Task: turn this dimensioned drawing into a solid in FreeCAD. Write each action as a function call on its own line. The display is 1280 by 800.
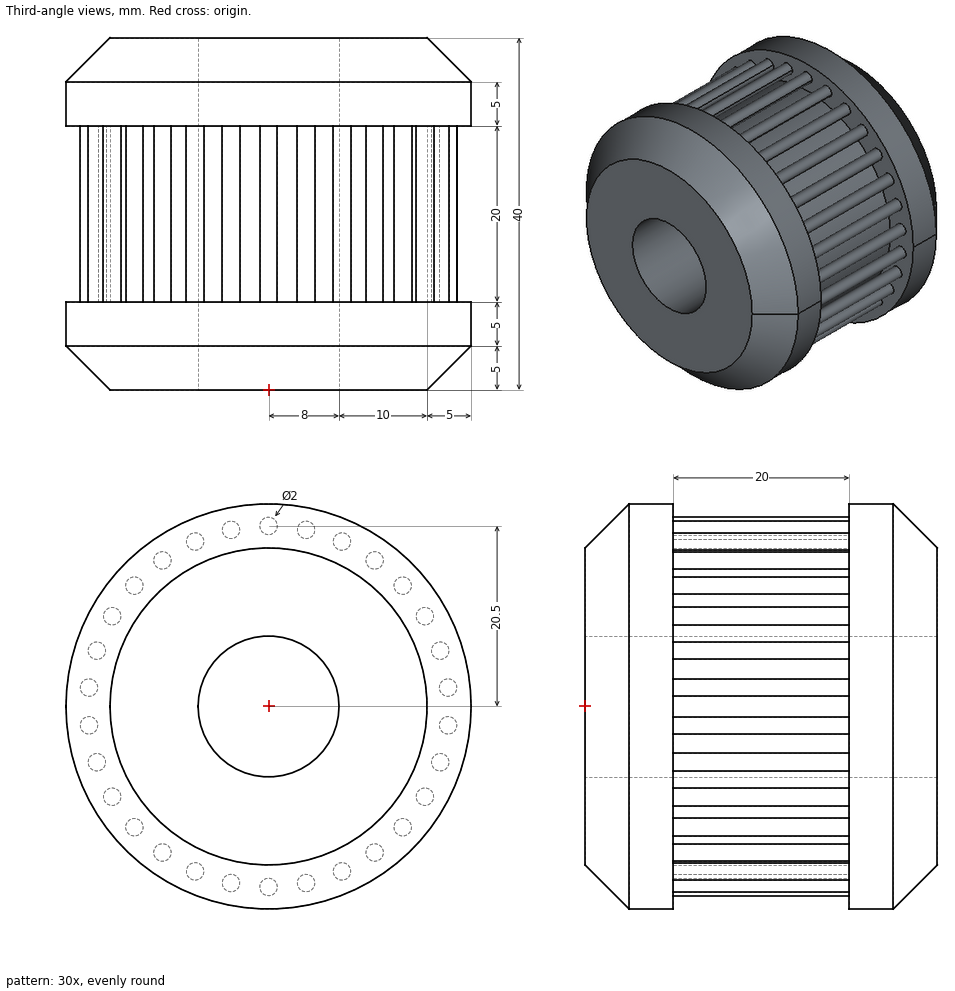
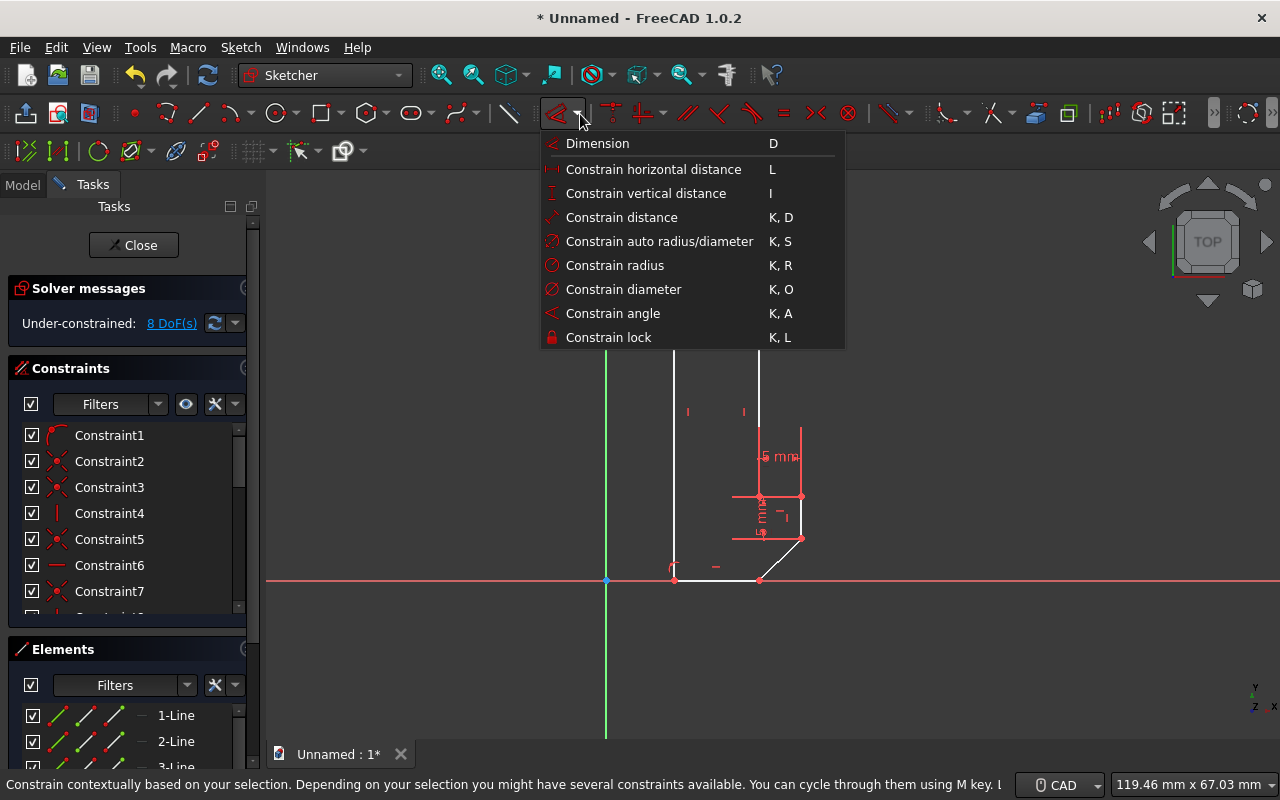
click(693, 193)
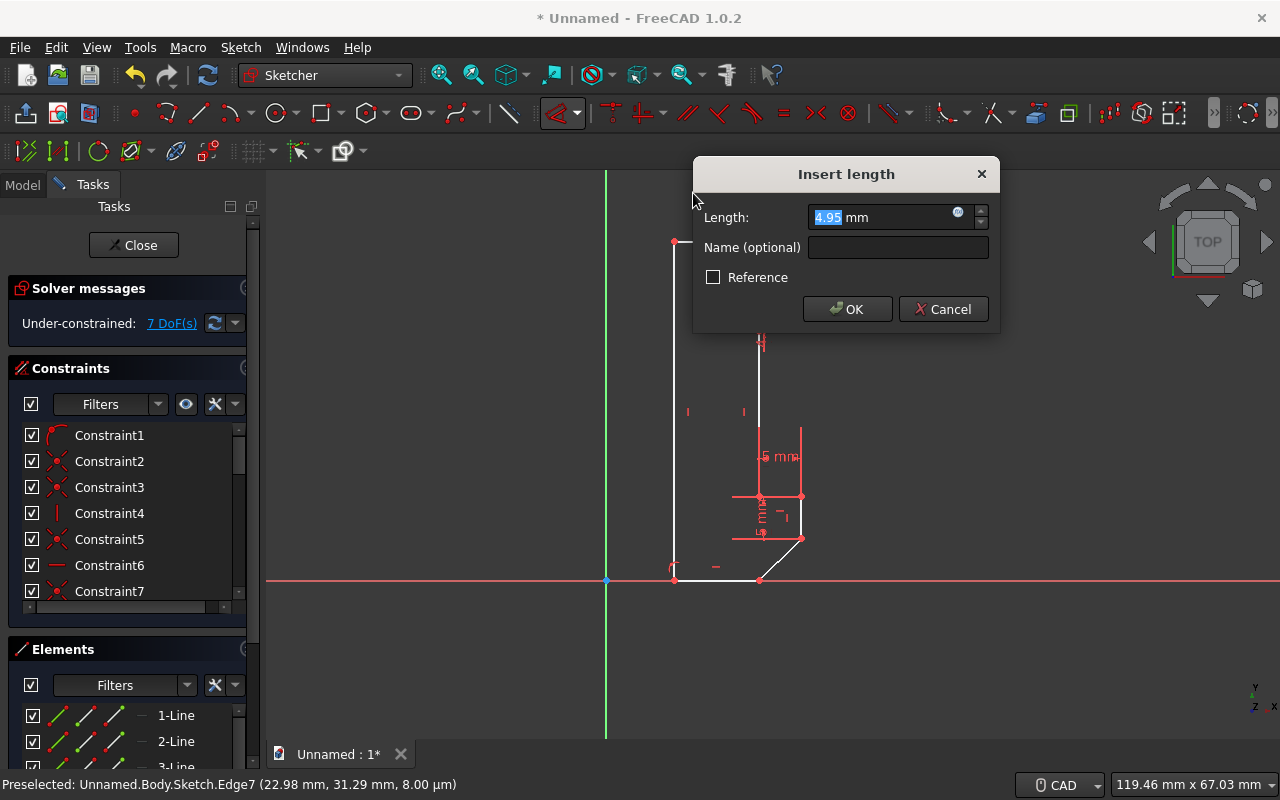
text(5)
key(Return)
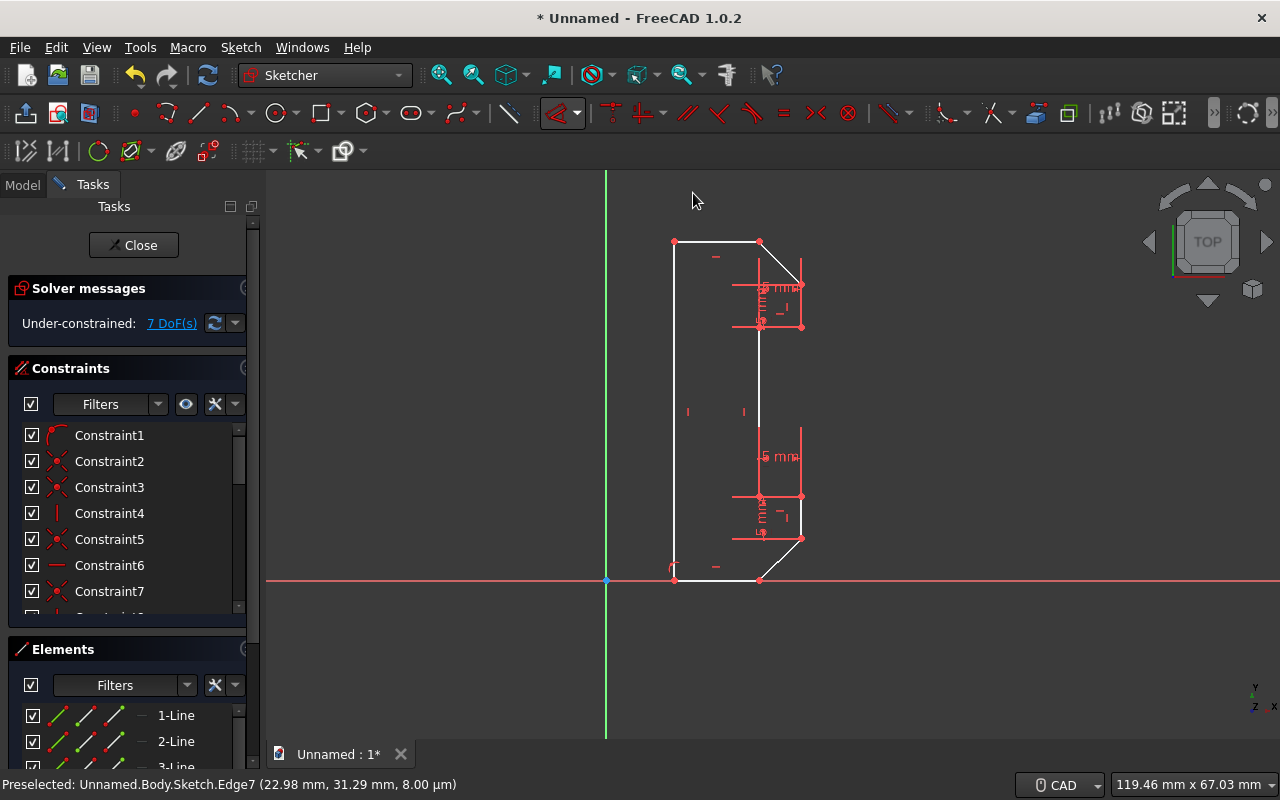
click(700, 581)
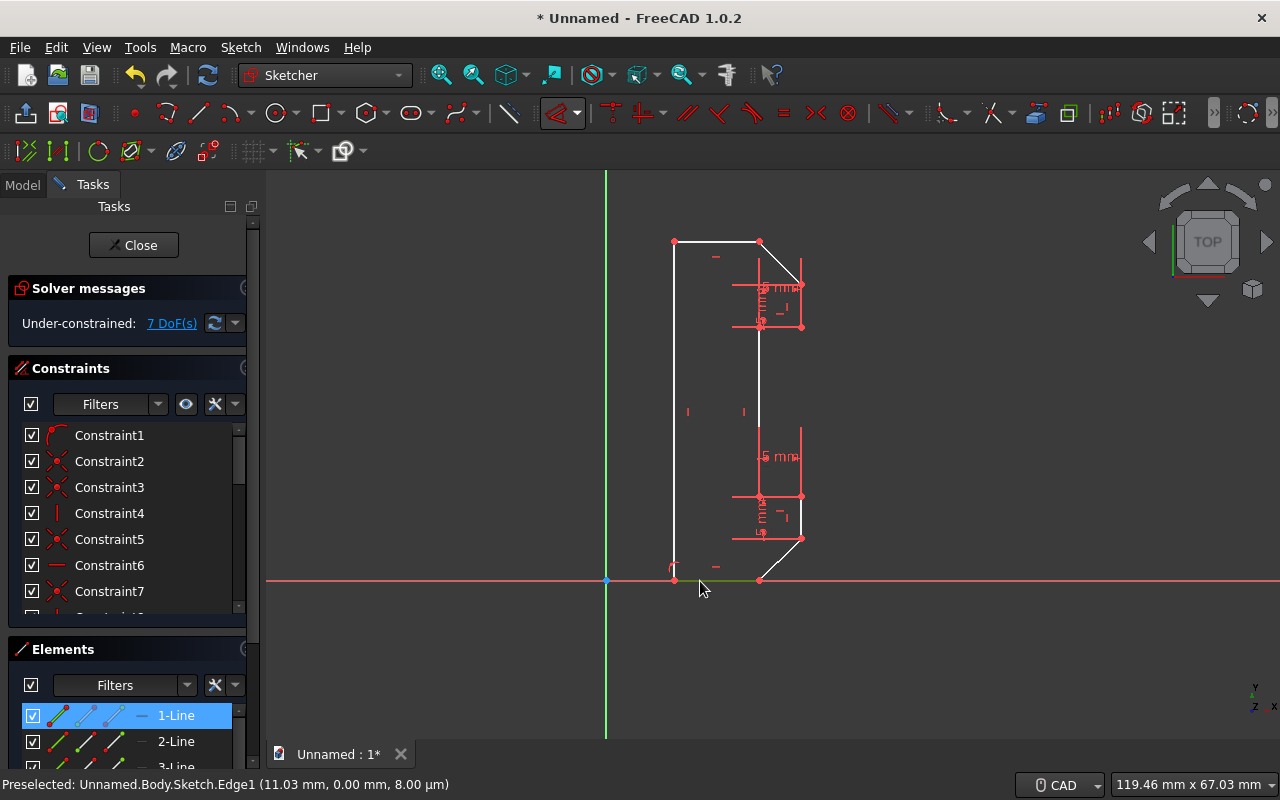
click(580, 114)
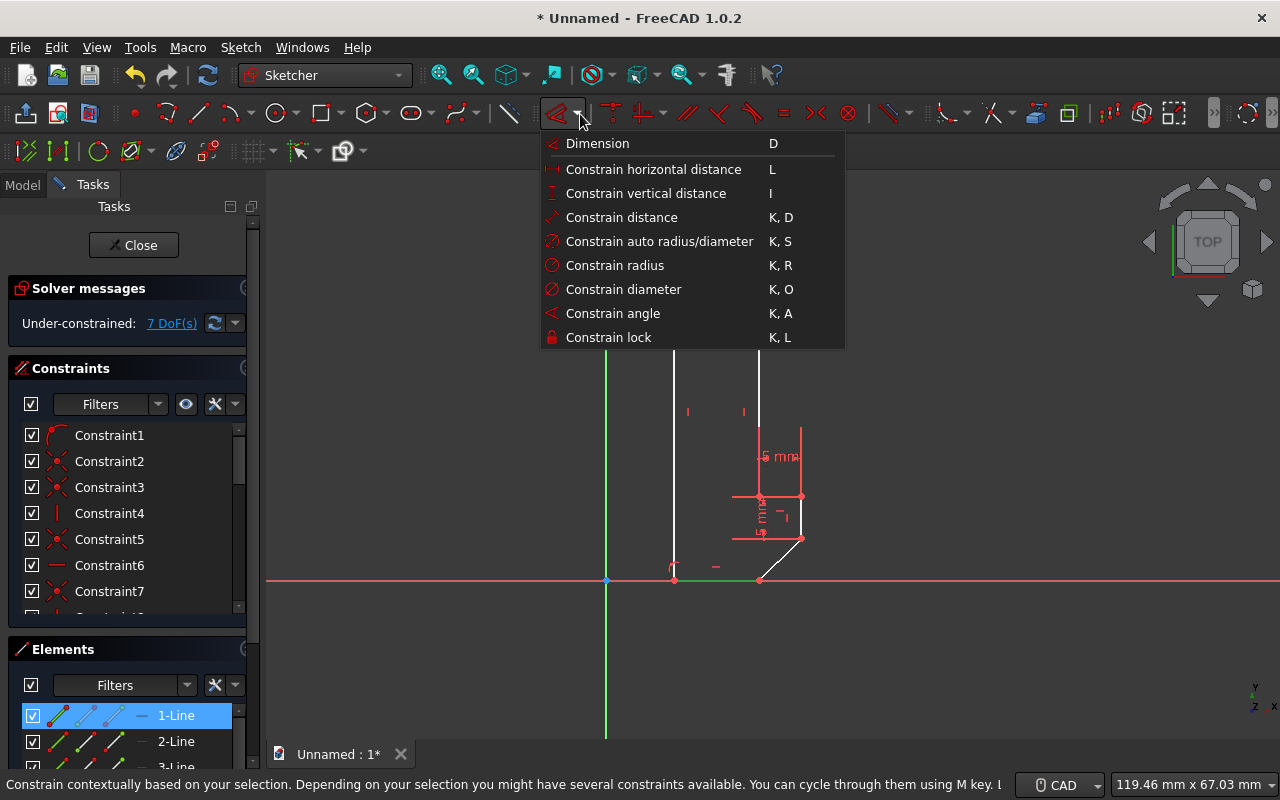
click(693, 169)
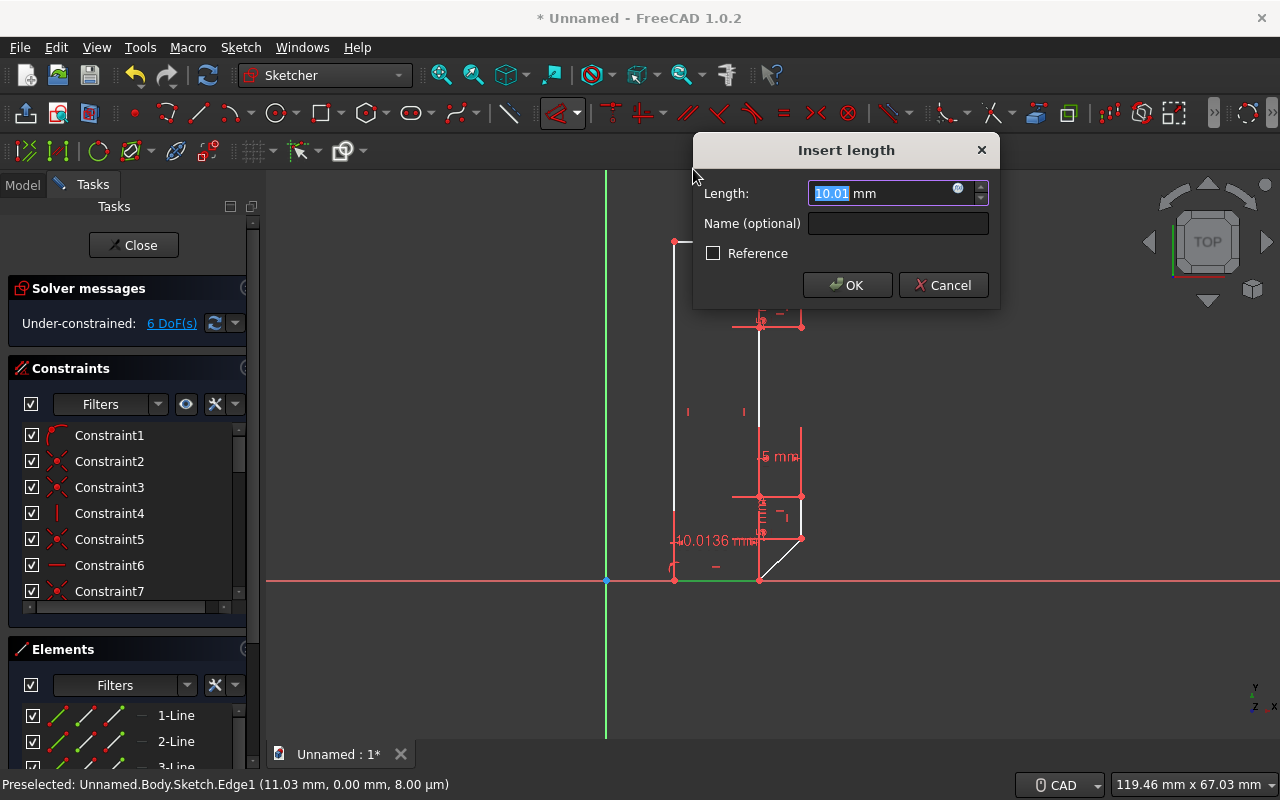
text(10)
key(Return)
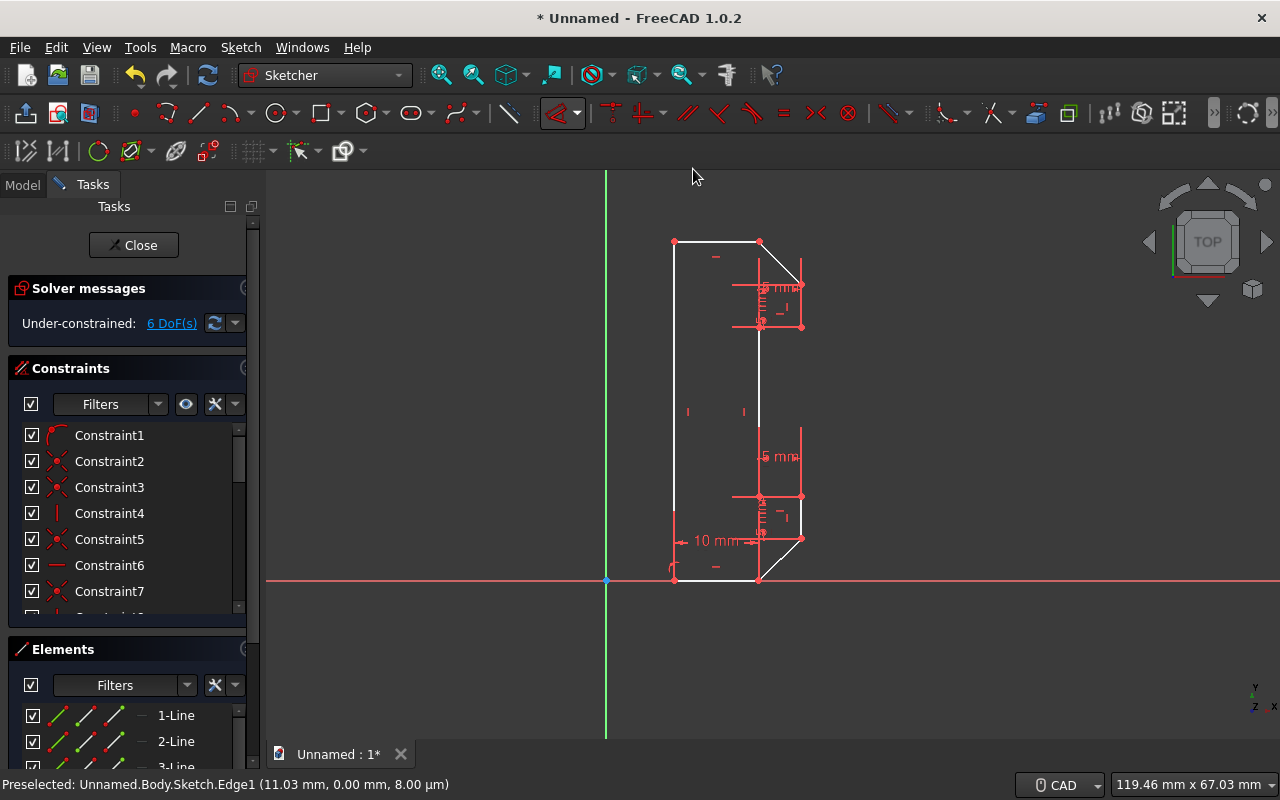
click(759, 446)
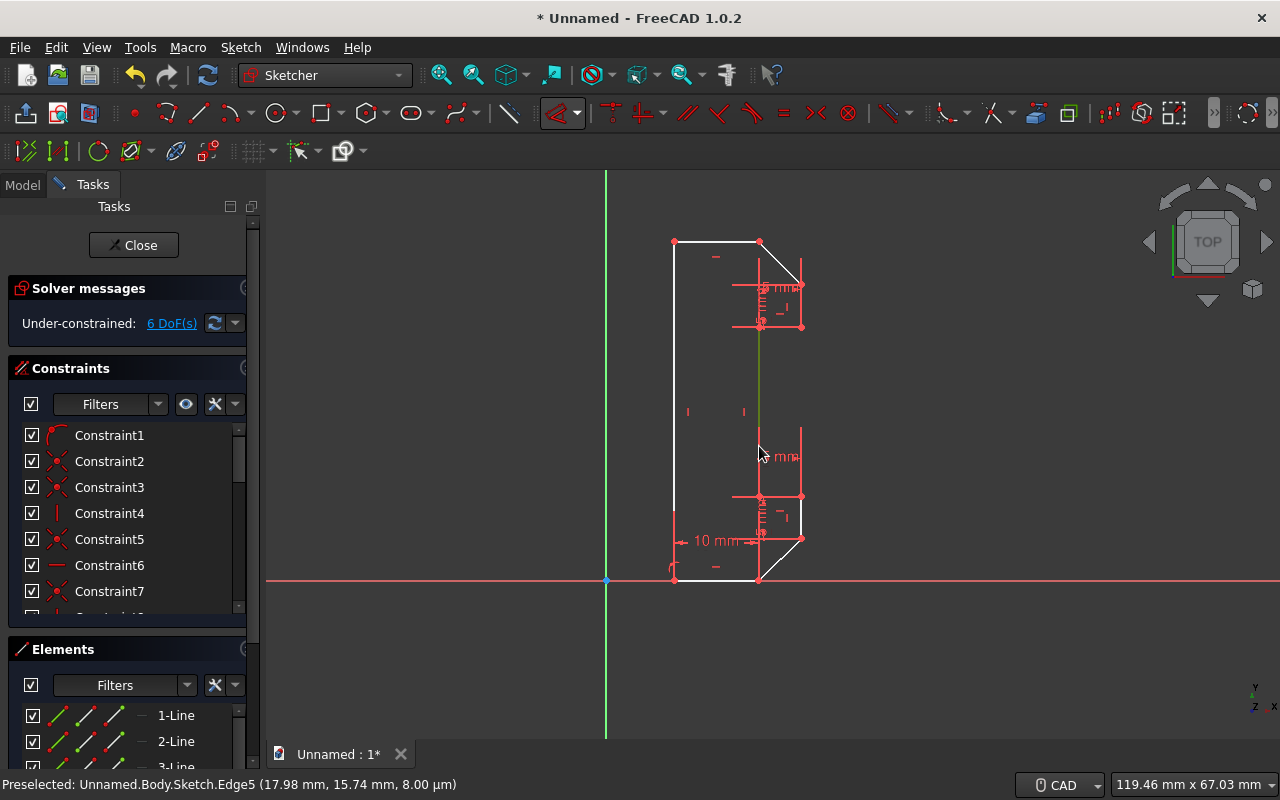
key(i)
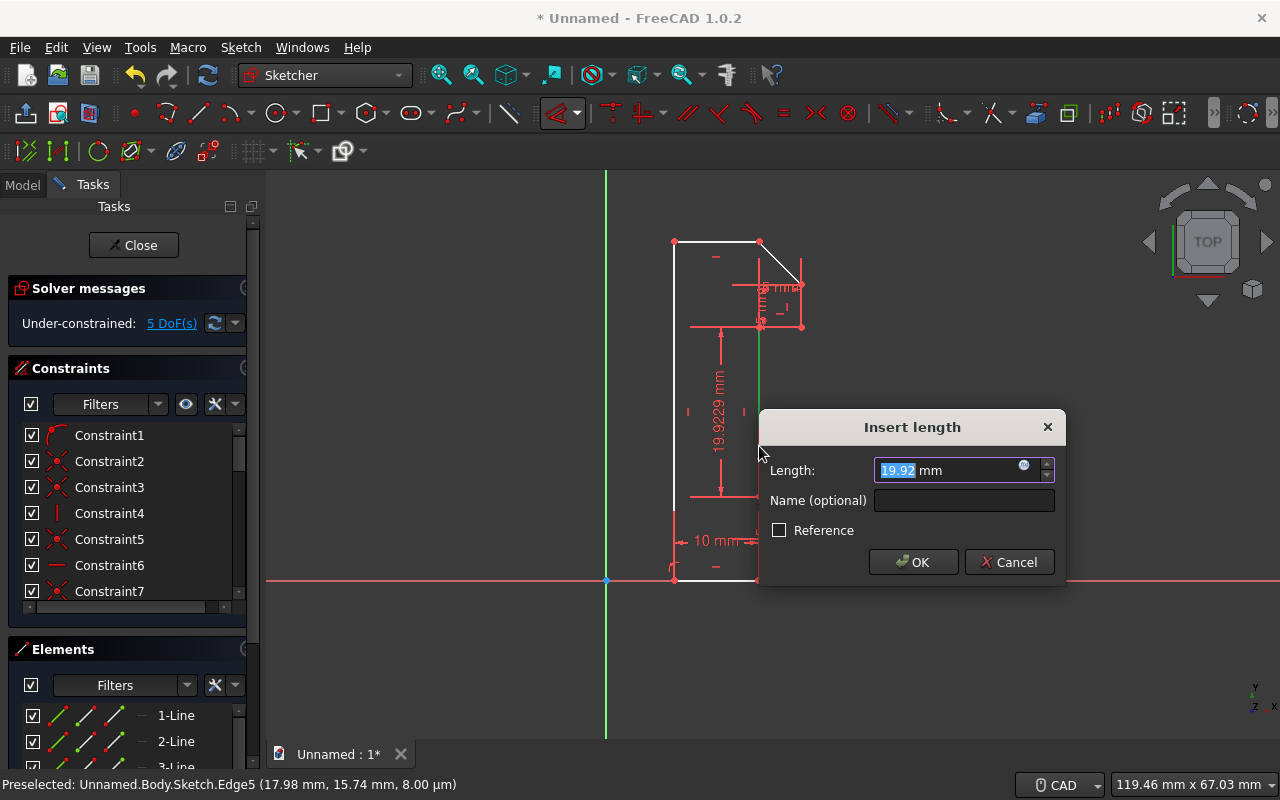
text(20)
key(Return)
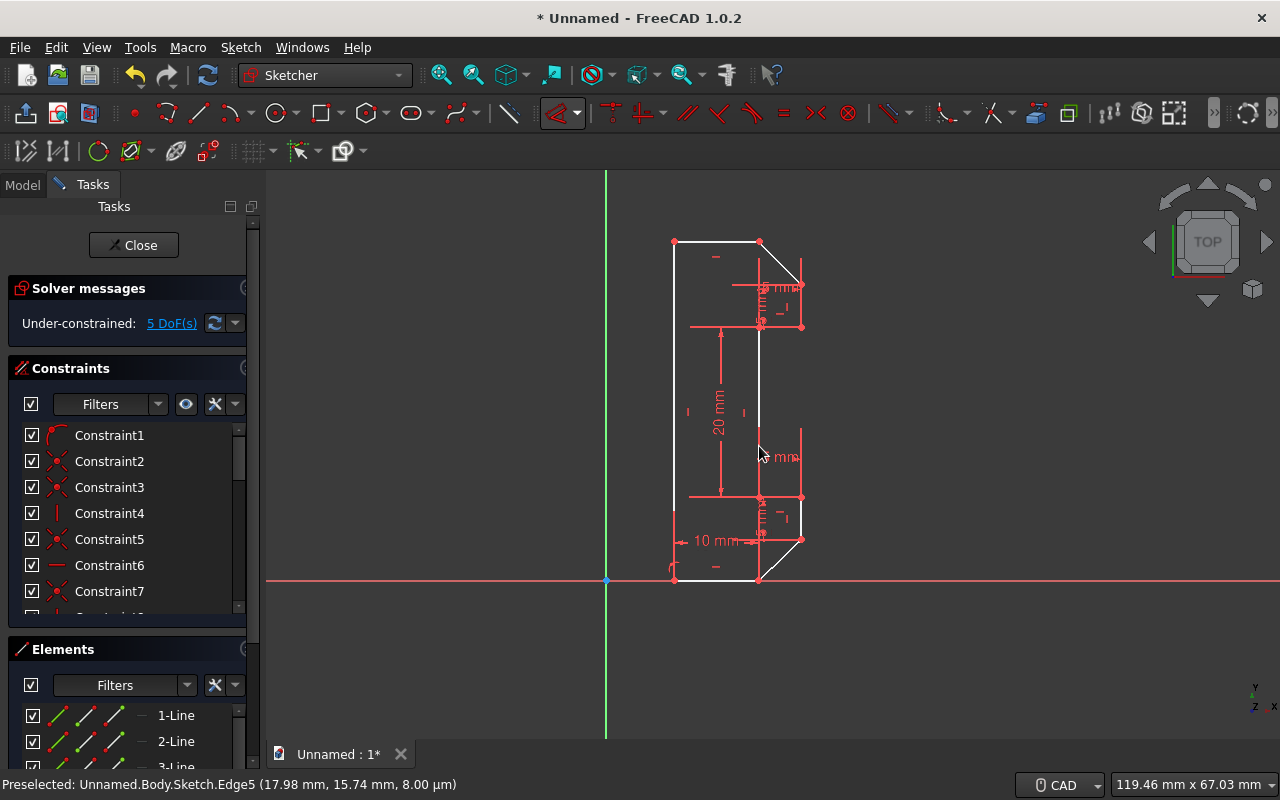
click(734, 242)